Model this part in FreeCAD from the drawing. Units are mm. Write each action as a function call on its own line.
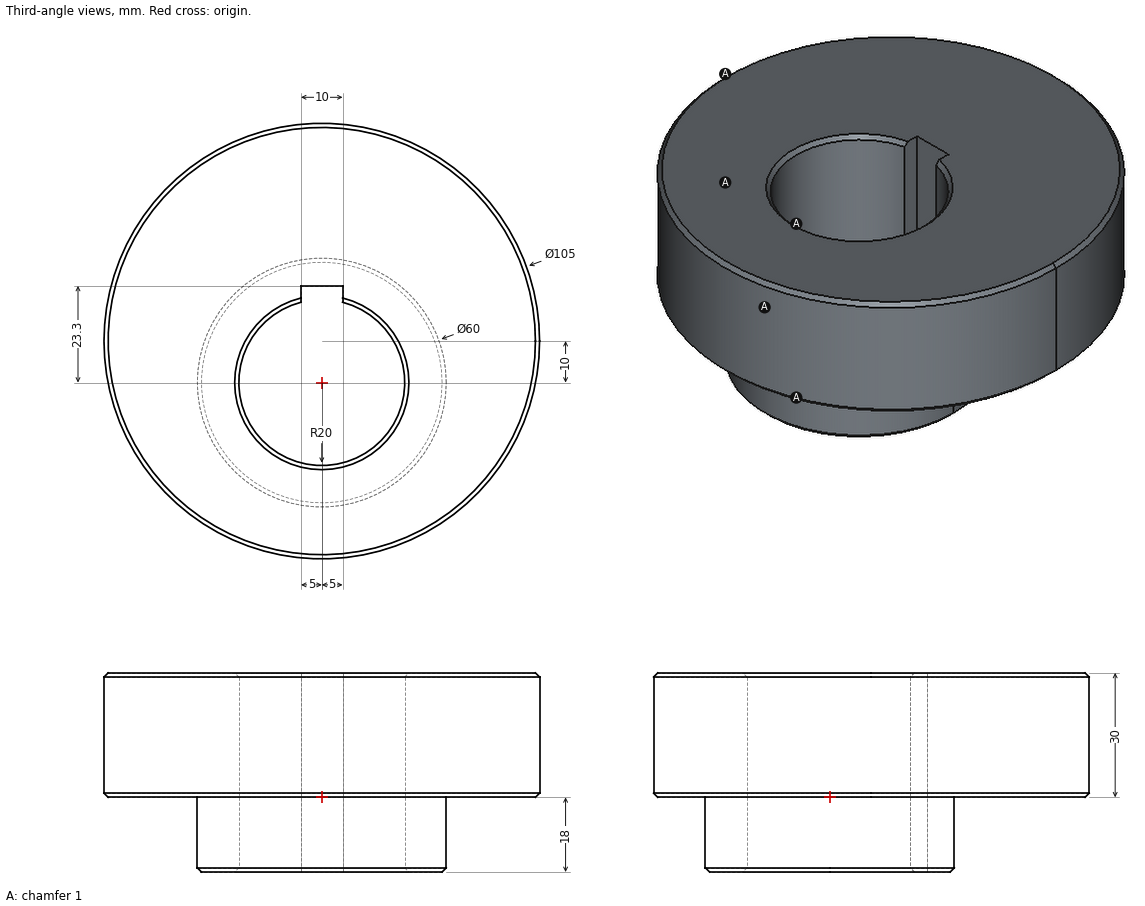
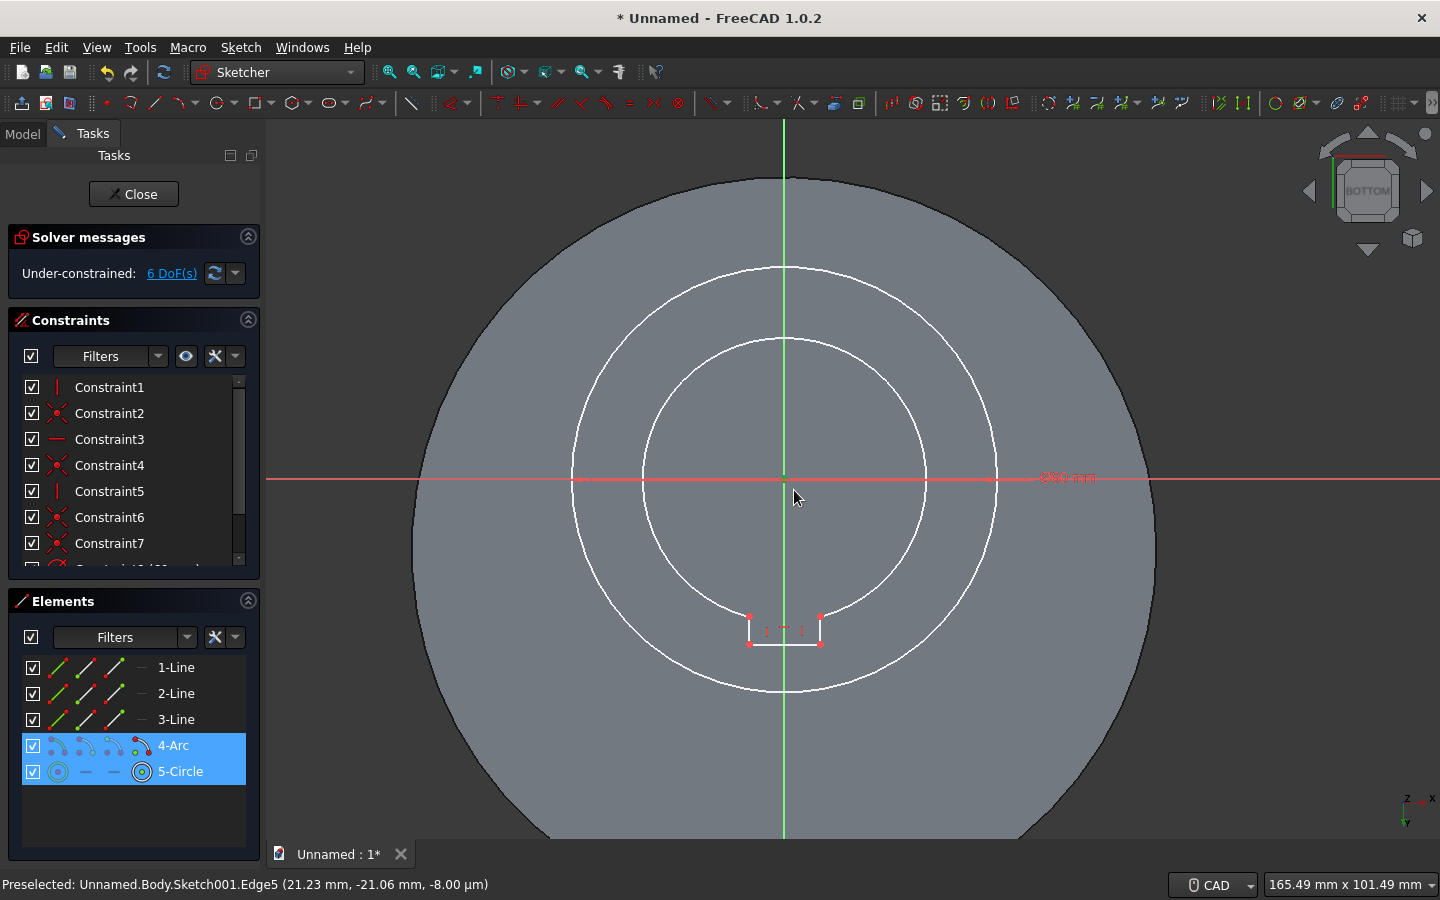
click(498, 104)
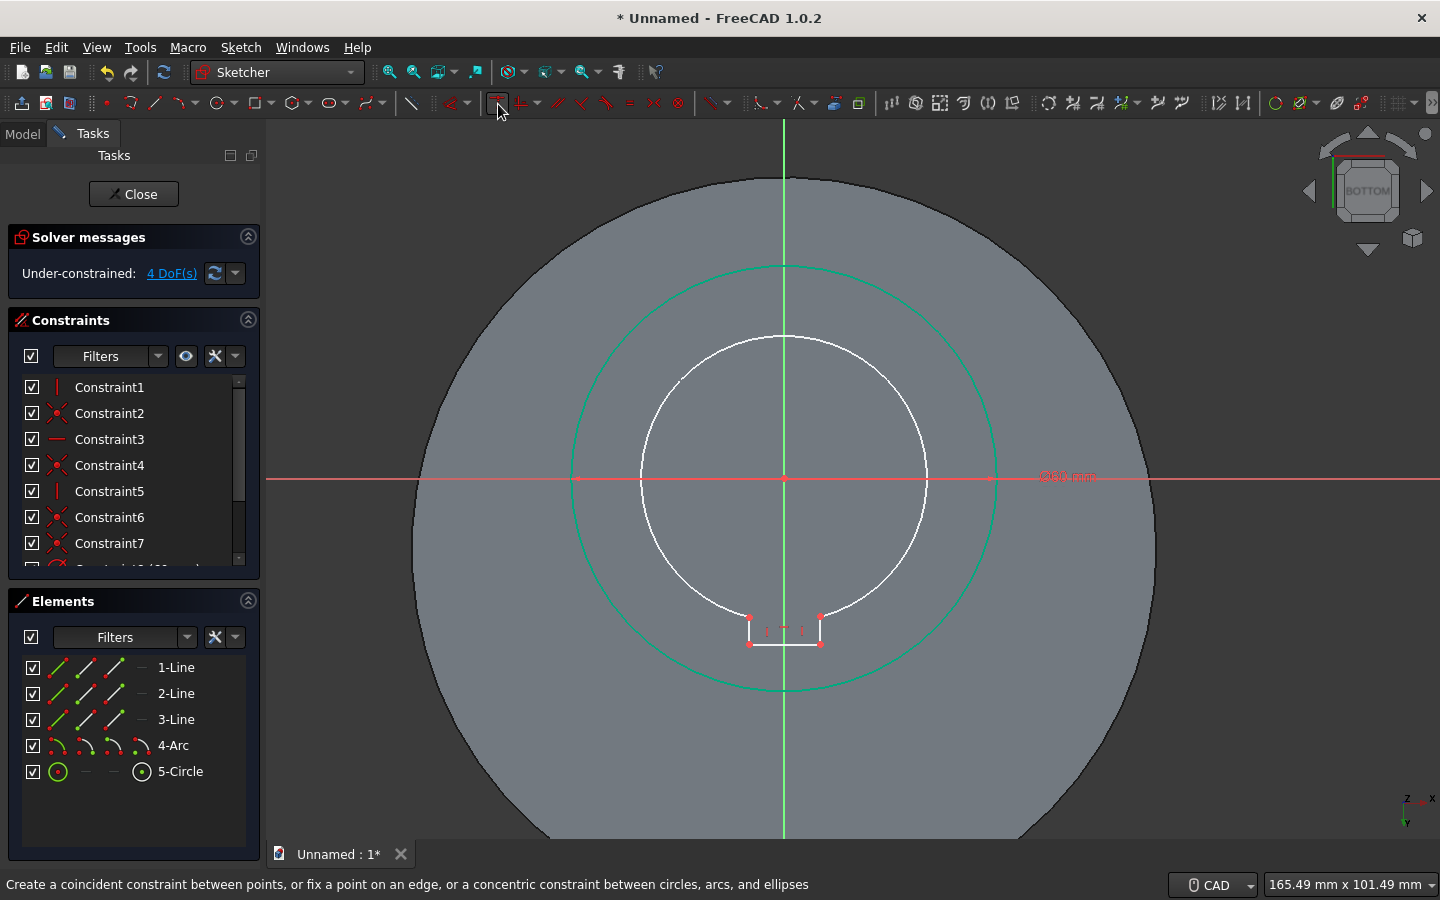
click(450, 104)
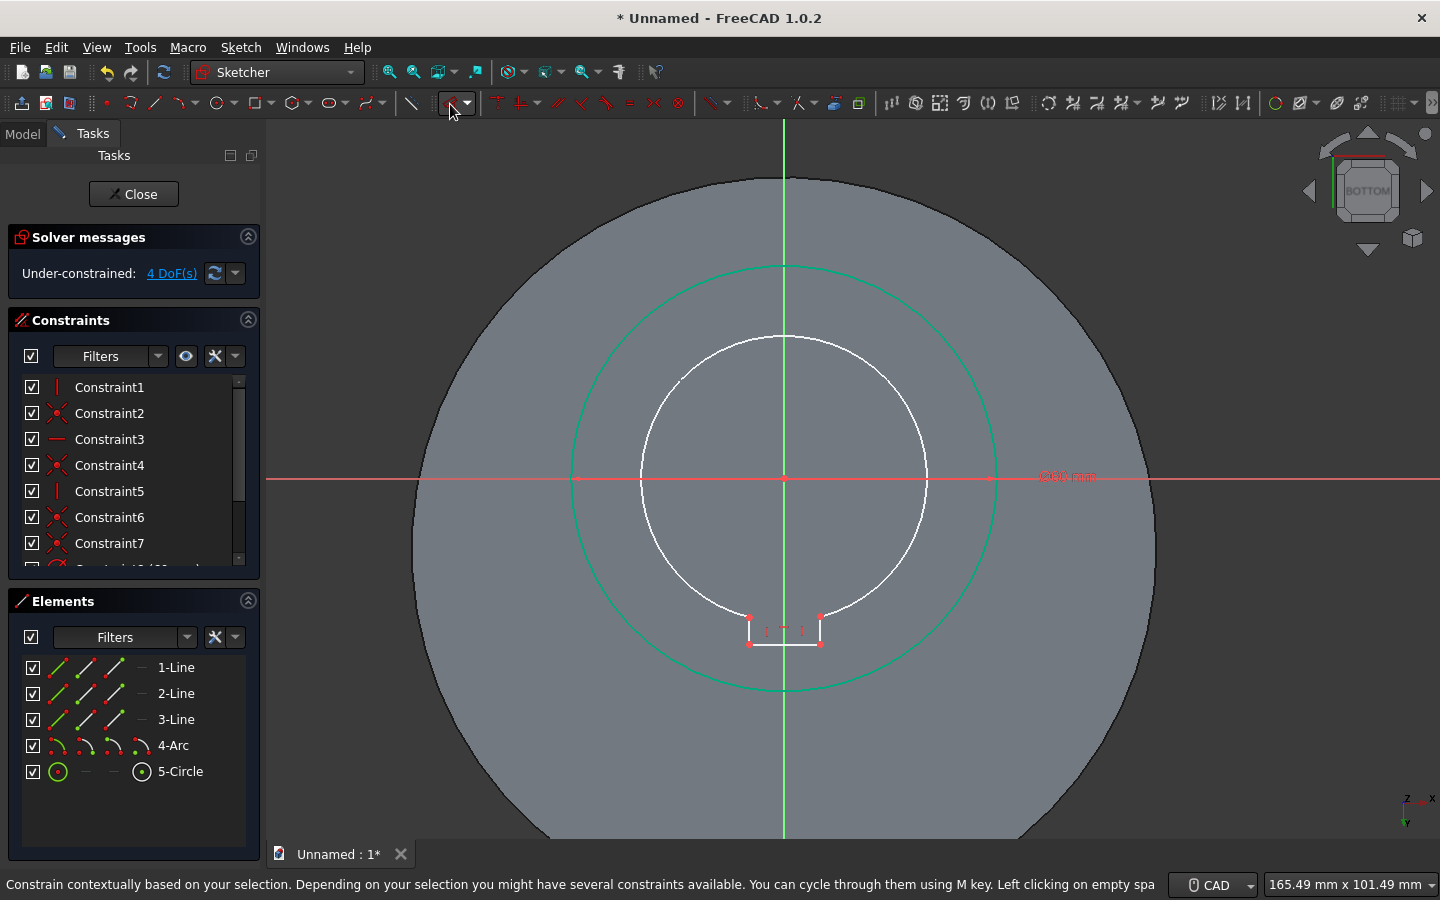
click(915, 421)
click(944, 408)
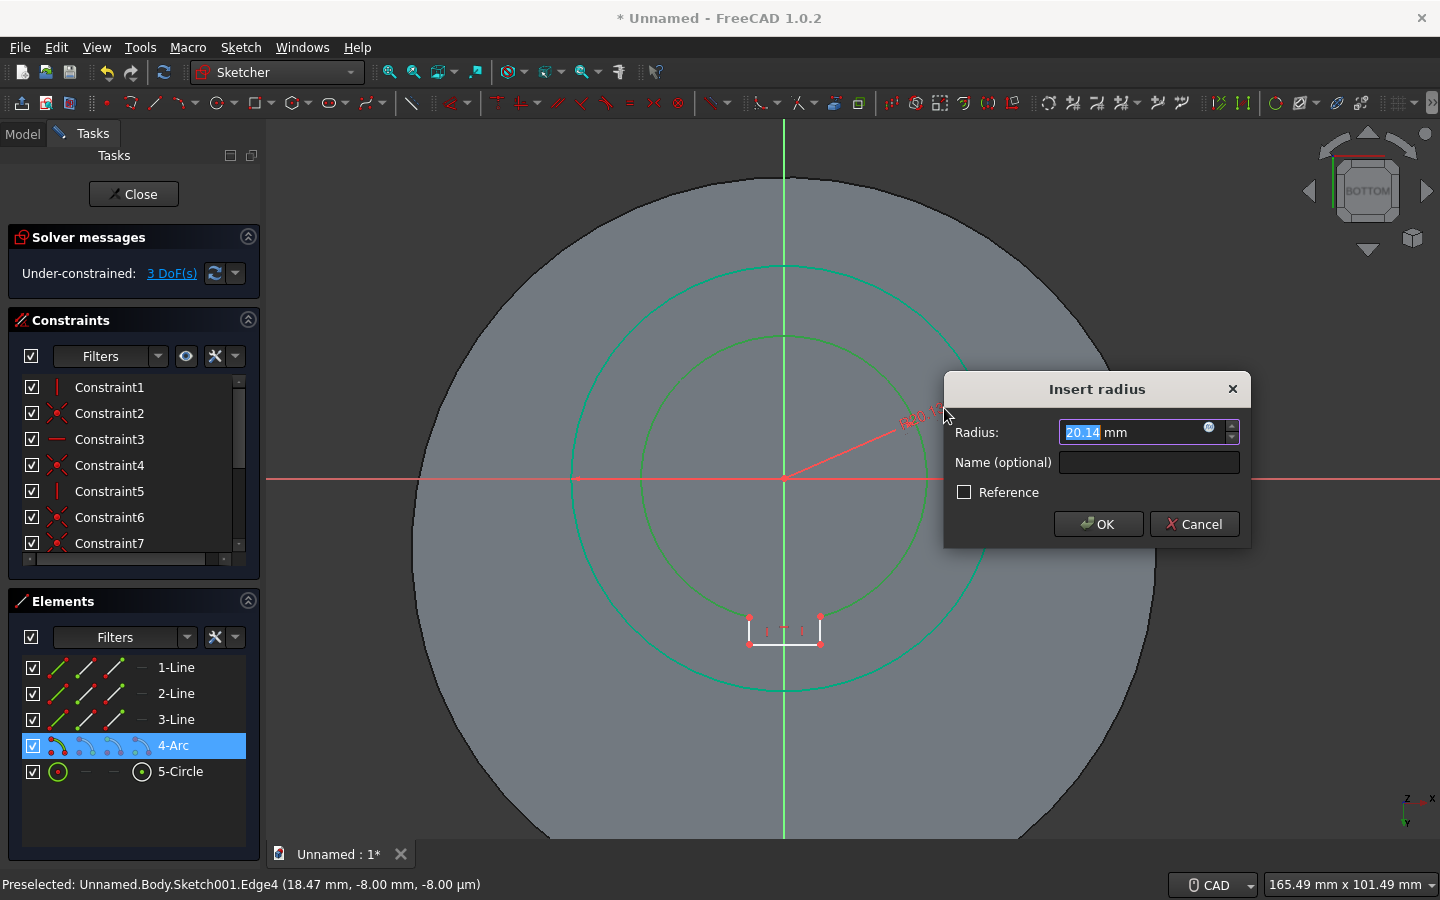
text(20)
key(Return)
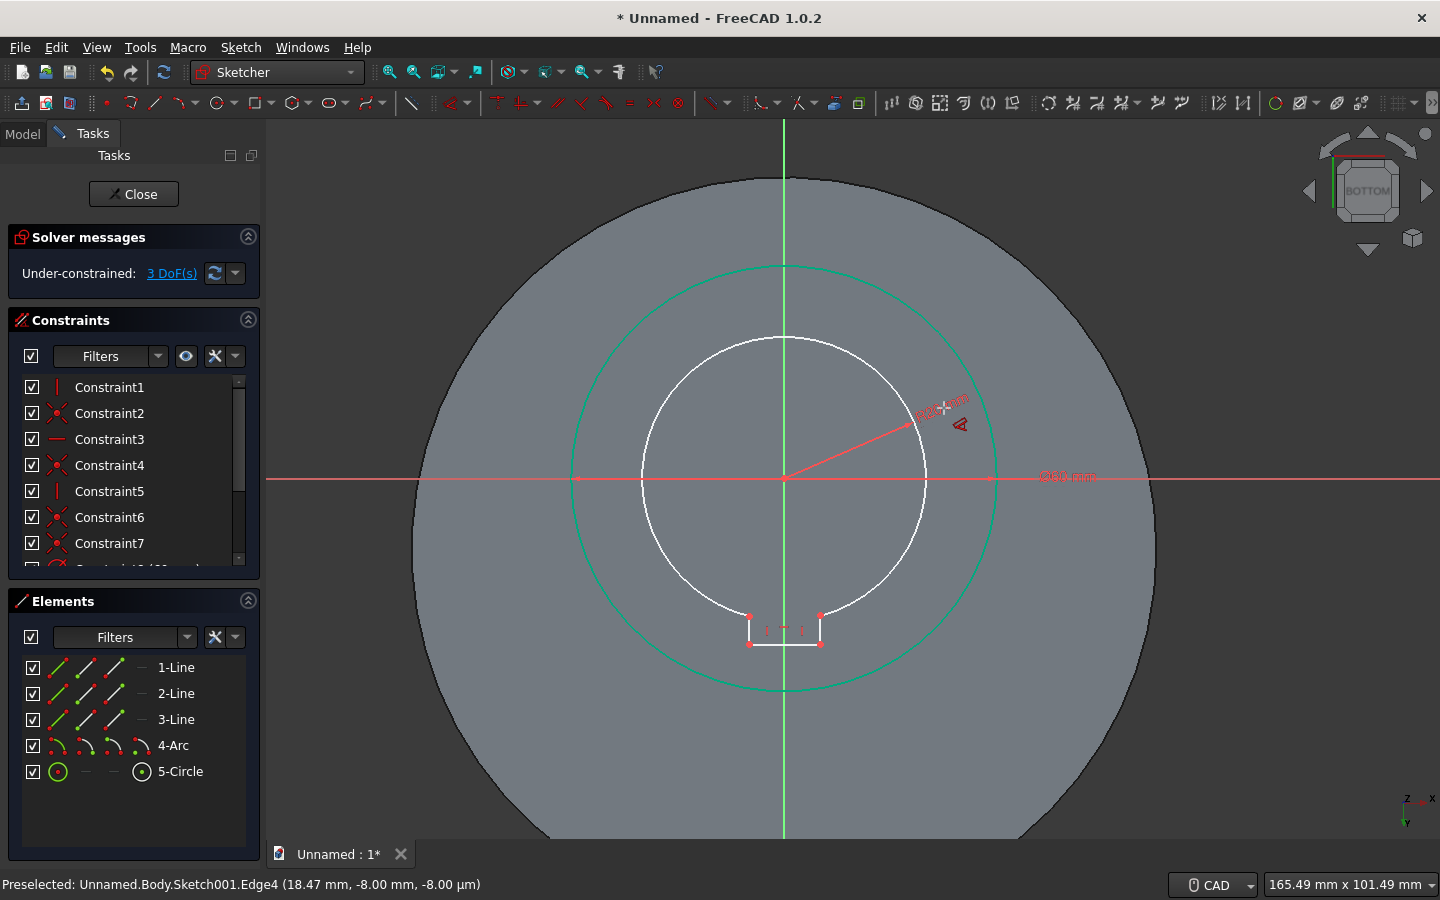
click(770, 645)
click(768, 611)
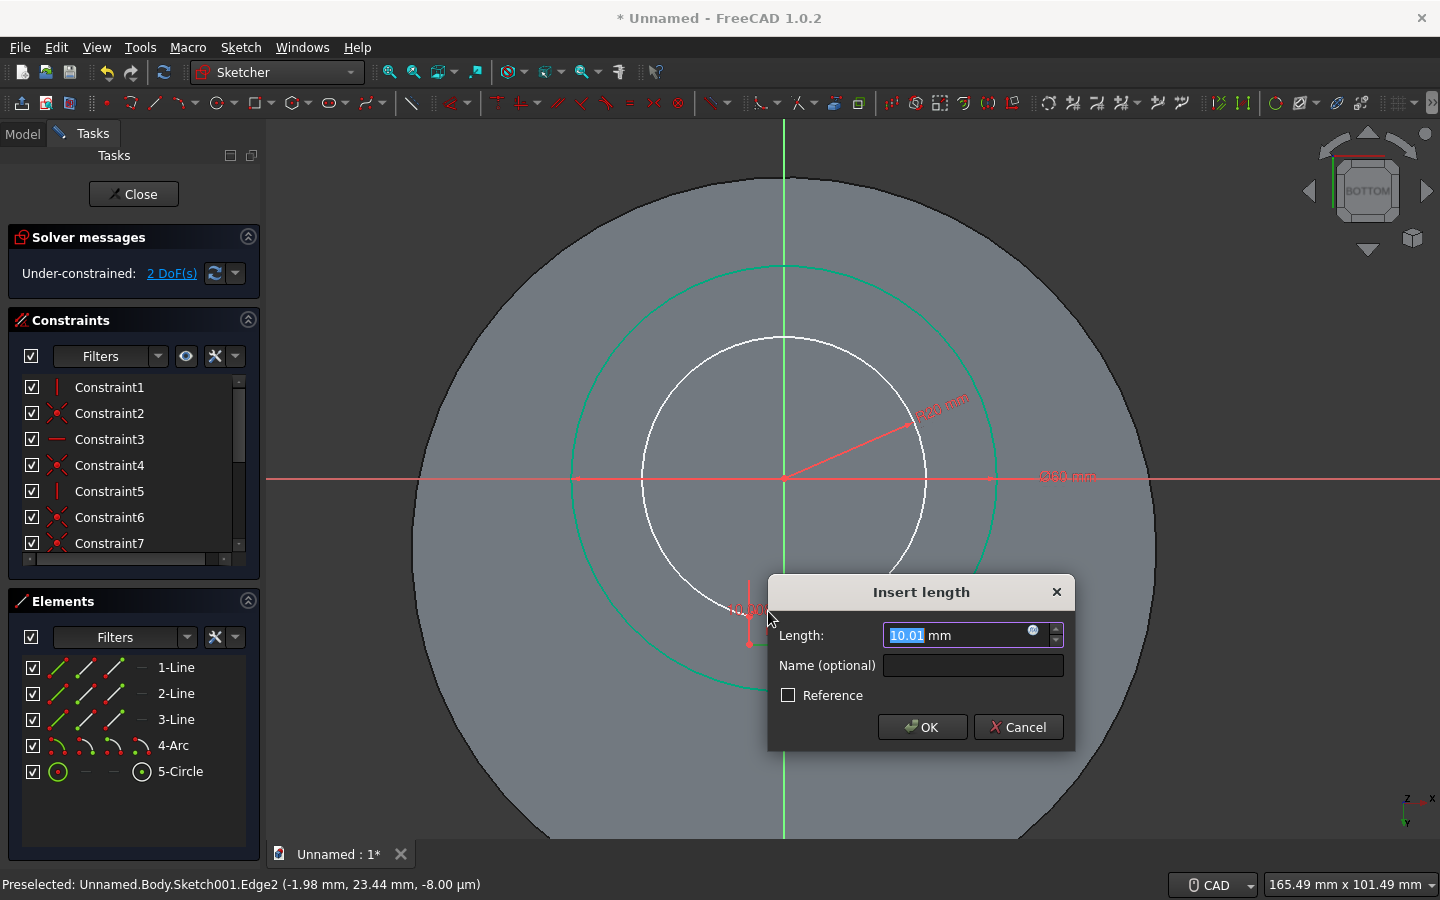
text(10)
key(Return)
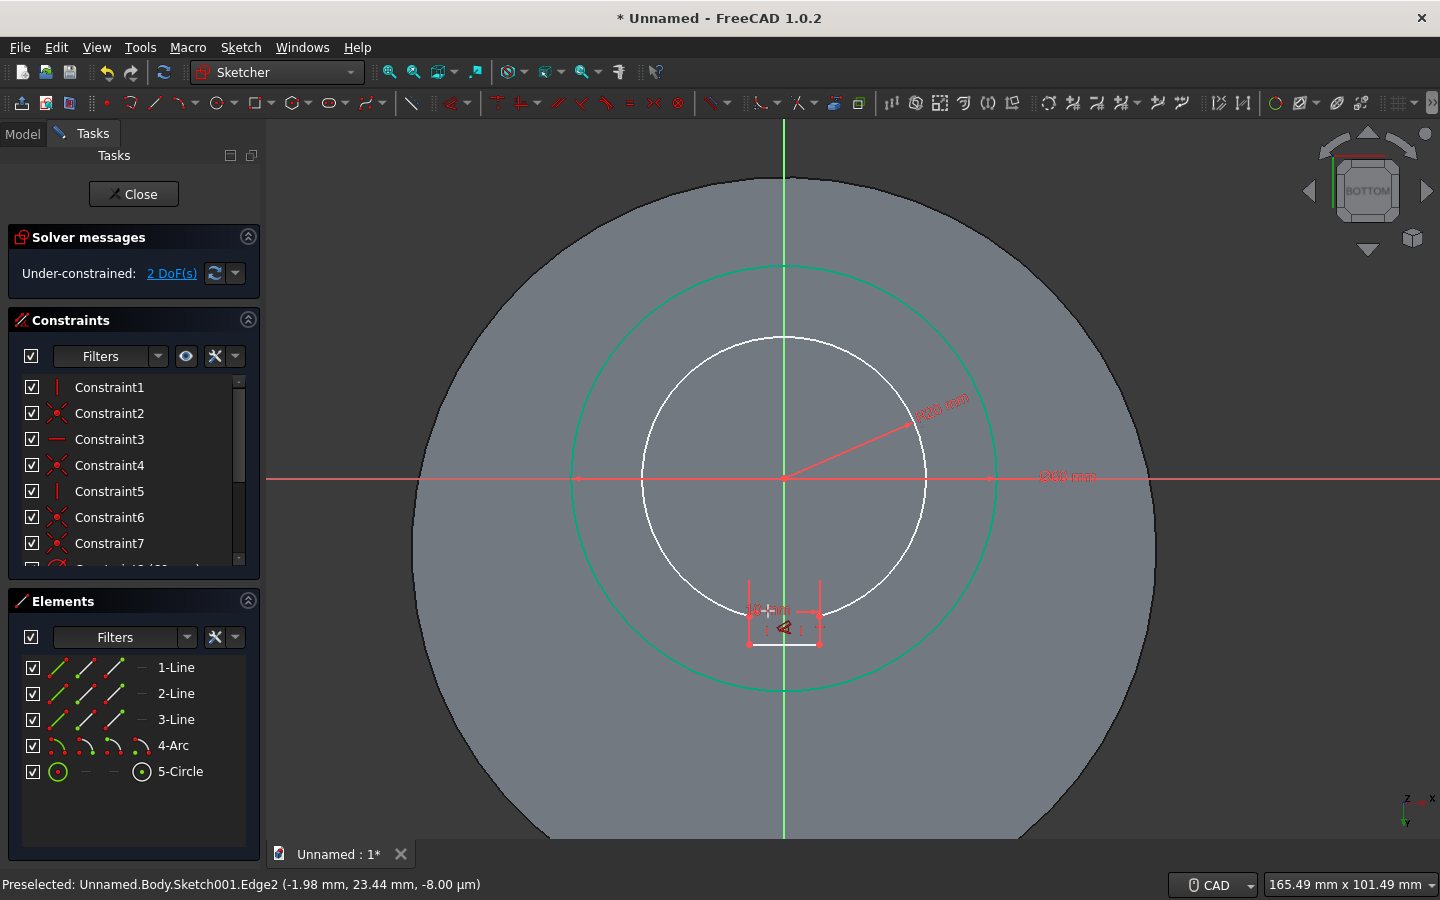
click(749, 616)
click(767, 445)